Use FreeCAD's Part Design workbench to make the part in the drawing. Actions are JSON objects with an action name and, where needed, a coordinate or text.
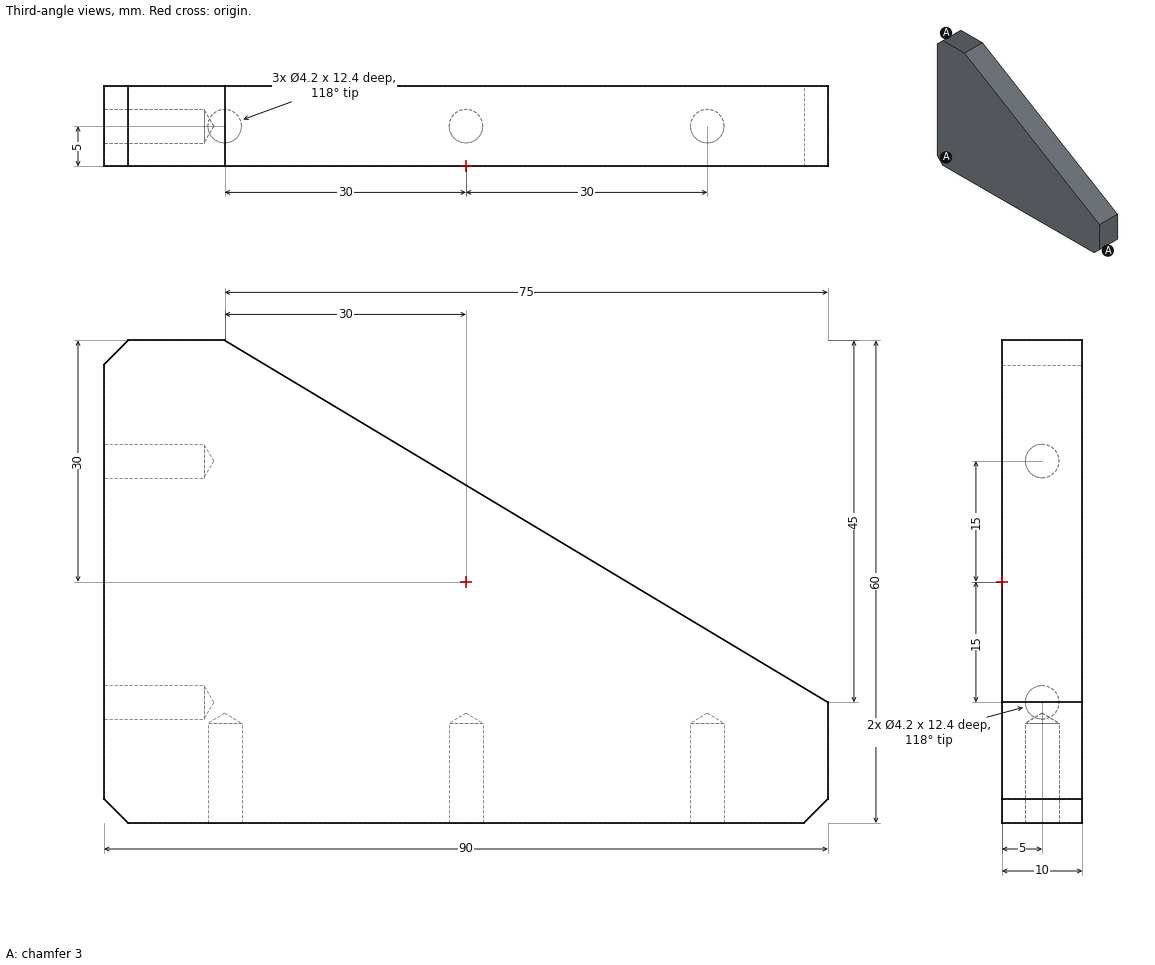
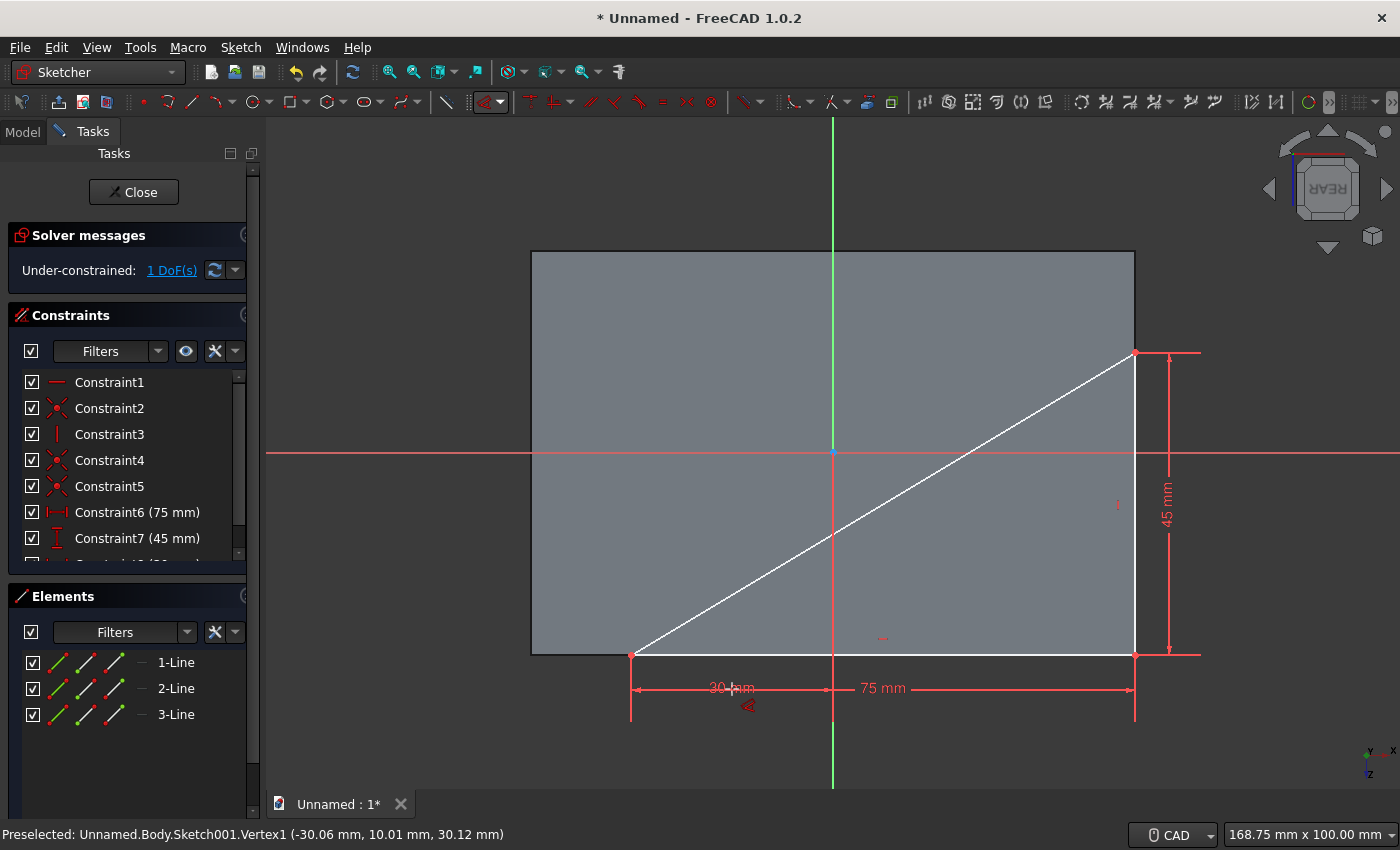
{"action": "left_click", "coordinate": [631, 655]}
{"action": "left_click", "coordinate": [597, 554]}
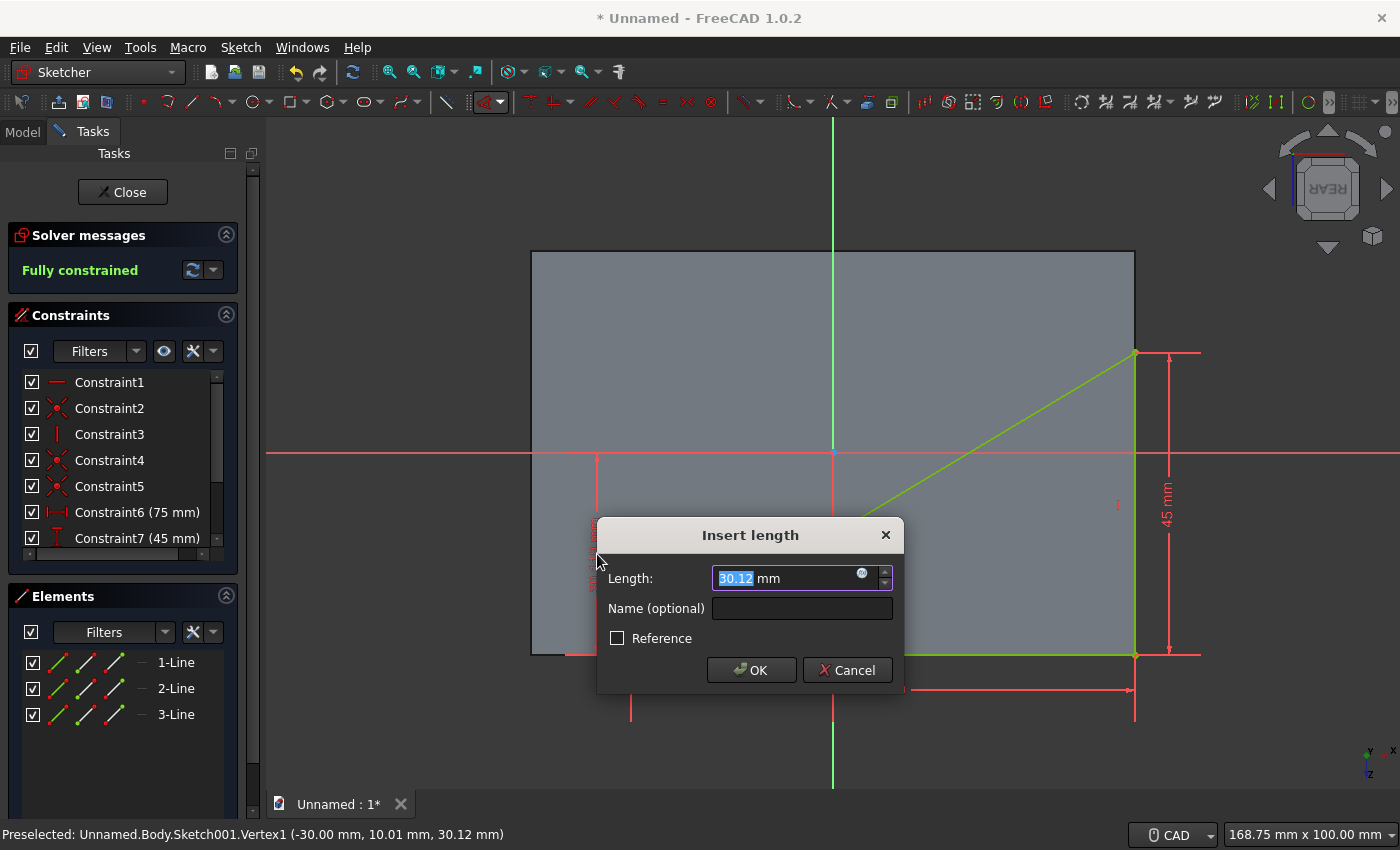
{"action": "type", "text": "30"}
{"action": "key", "text": "Return"}
{"action": "key", "text": "Escape"}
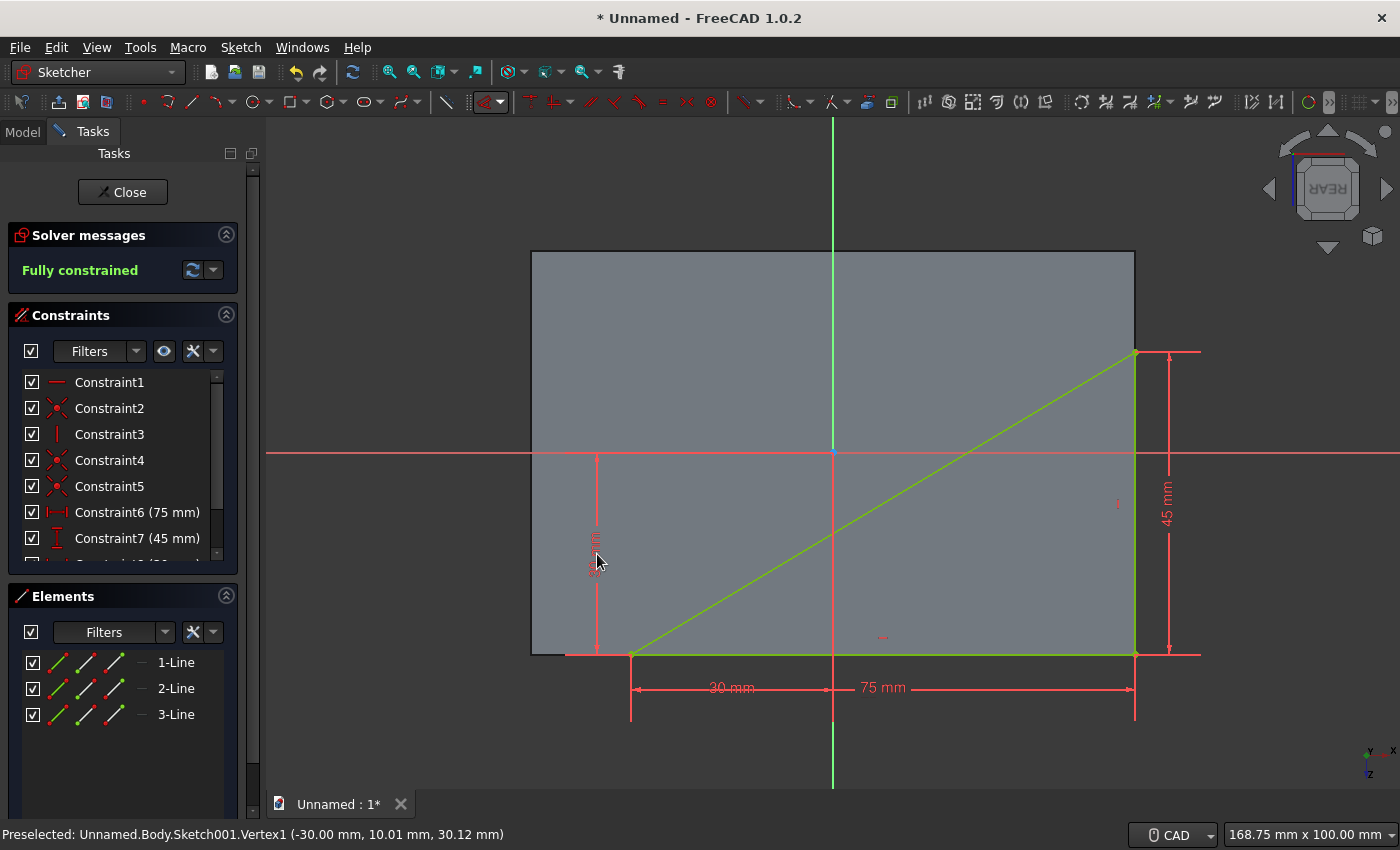
{"action": "left_click", "coordinate": [123, 192]}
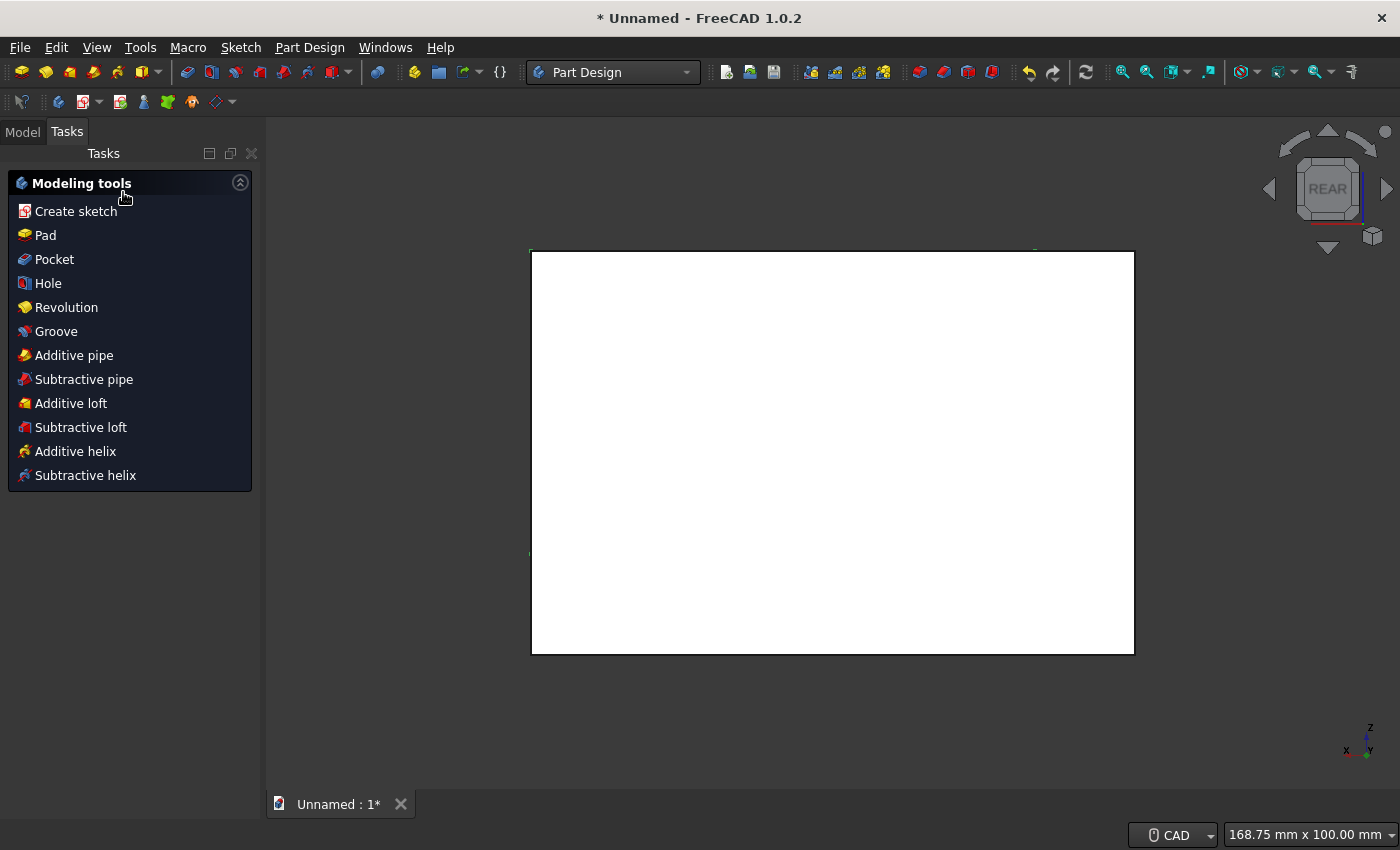
{"action": "left_click", "coordinate": [188, 72]}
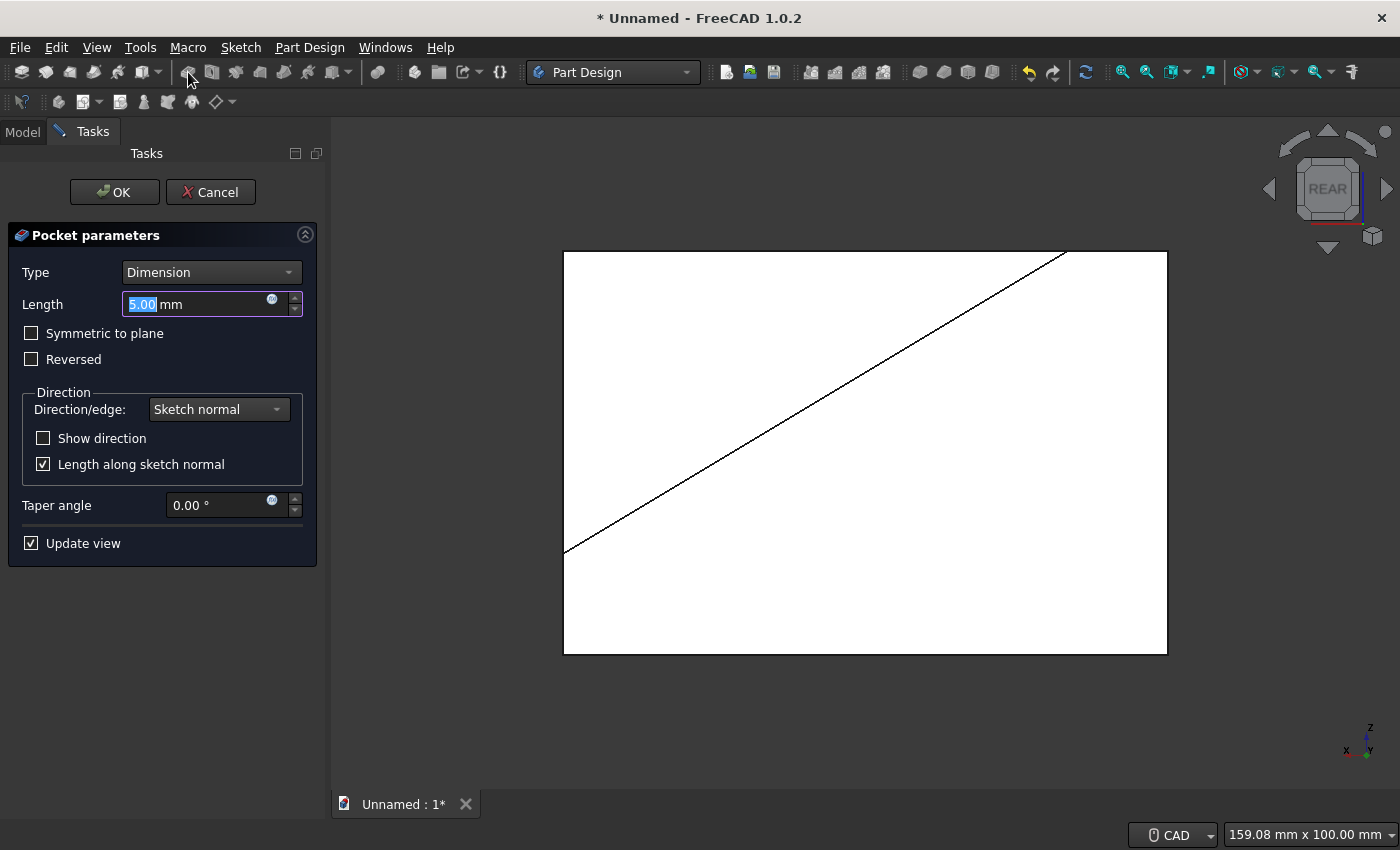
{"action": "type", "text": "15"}
{"action": "key", "text": "Tab"}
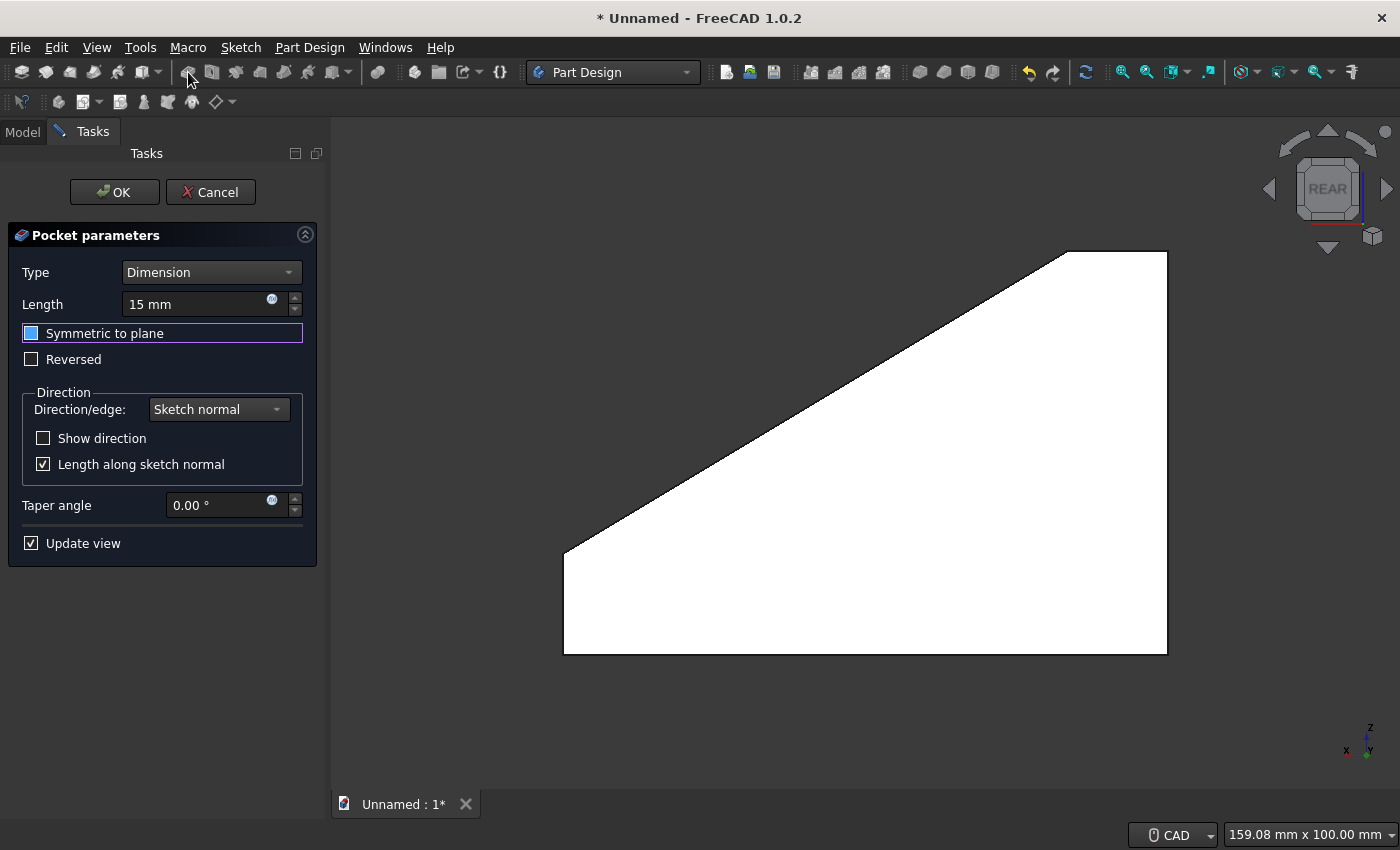
{"action": "left_click", "coordinate": [115, 192]}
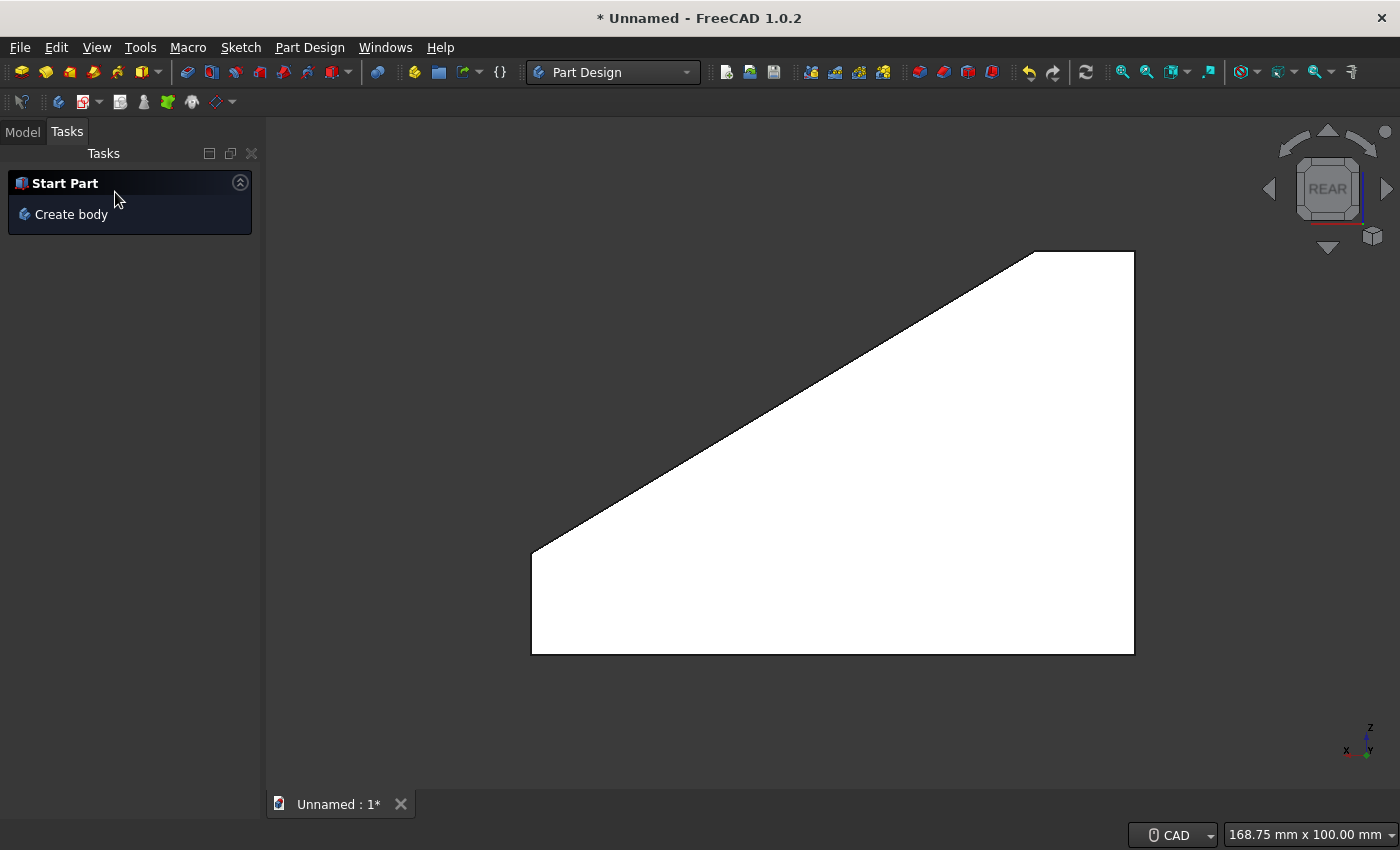
{"action": "key", "text": "0"}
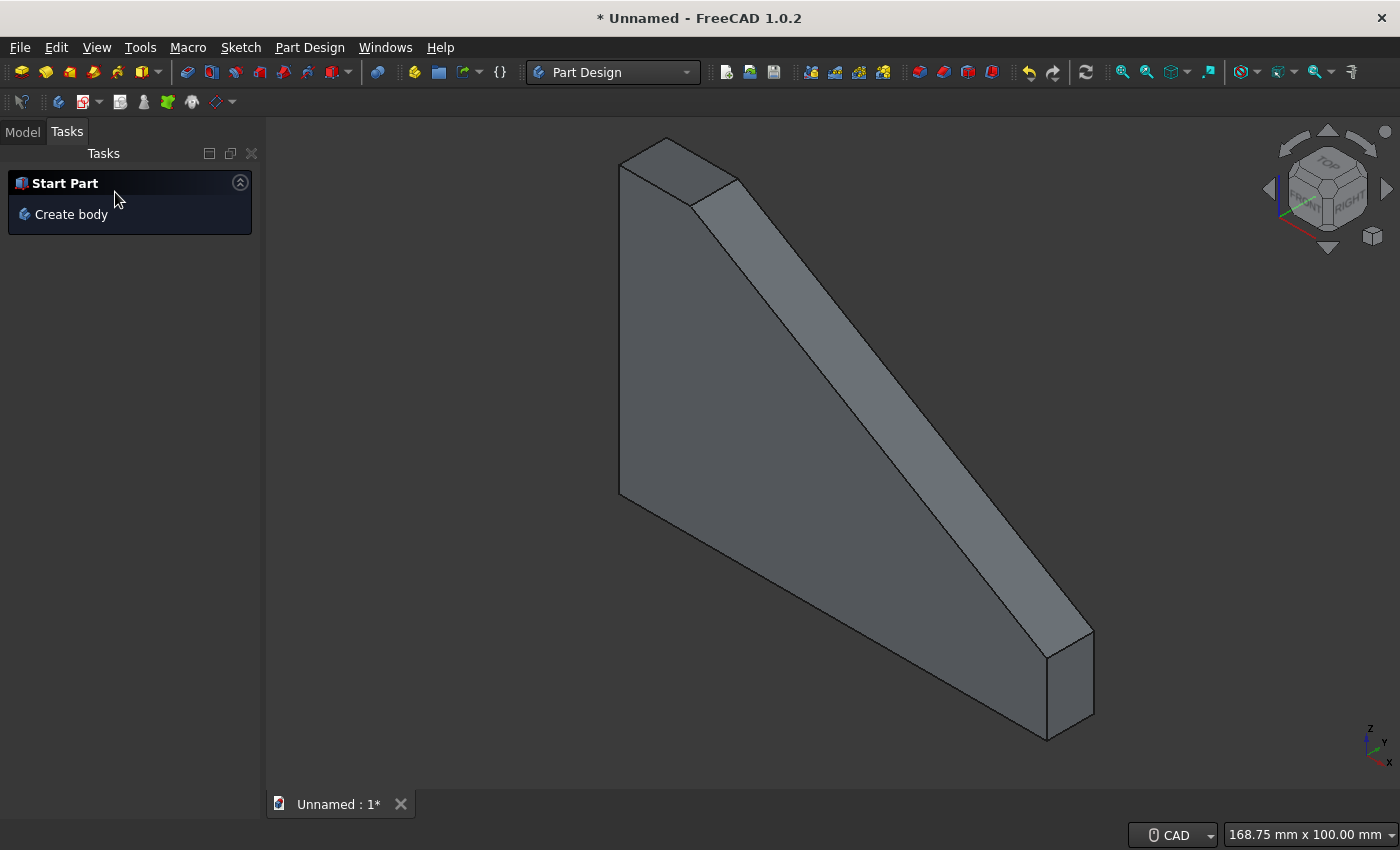
{"action": "key", "text": "2"}